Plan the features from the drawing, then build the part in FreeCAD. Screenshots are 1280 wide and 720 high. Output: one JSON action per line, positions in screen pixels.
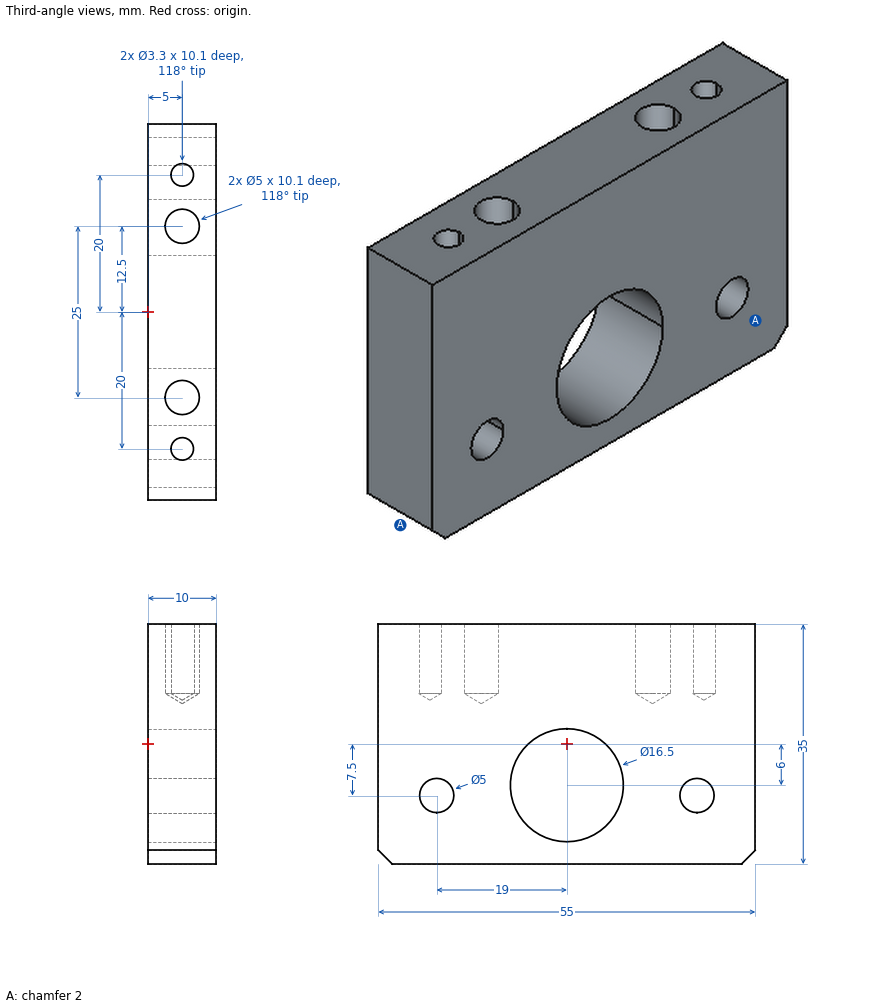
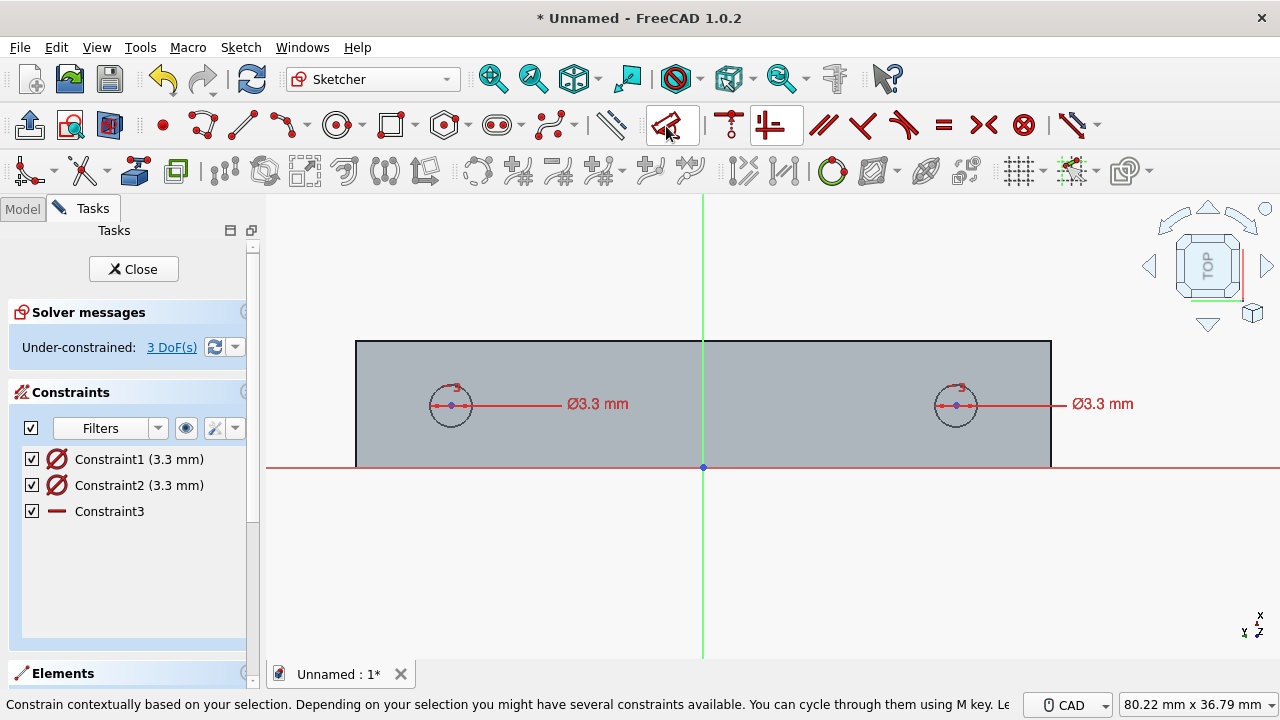
{"action": "left_click", "coordinate": [451, 406]}
{"action": "left_click", "coordinate": [417, 437]}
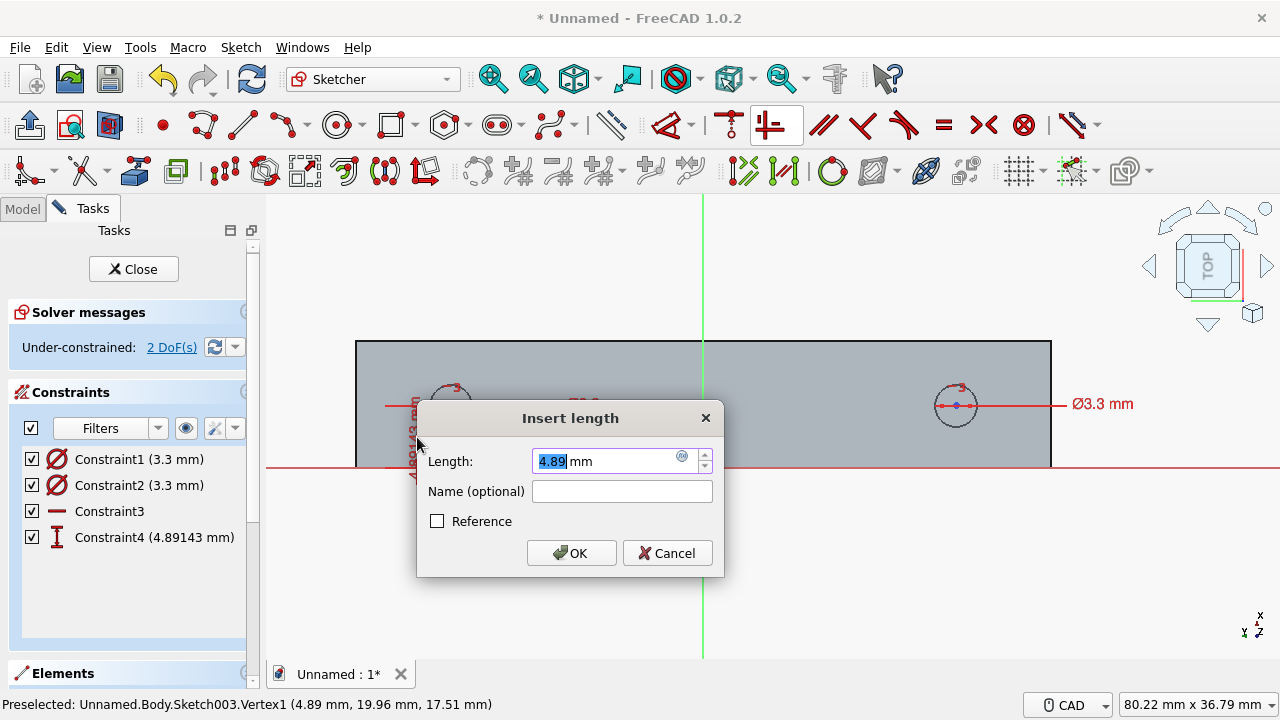
{"action": "type", "text": "5"}
{"action": "key", "text": "Return"}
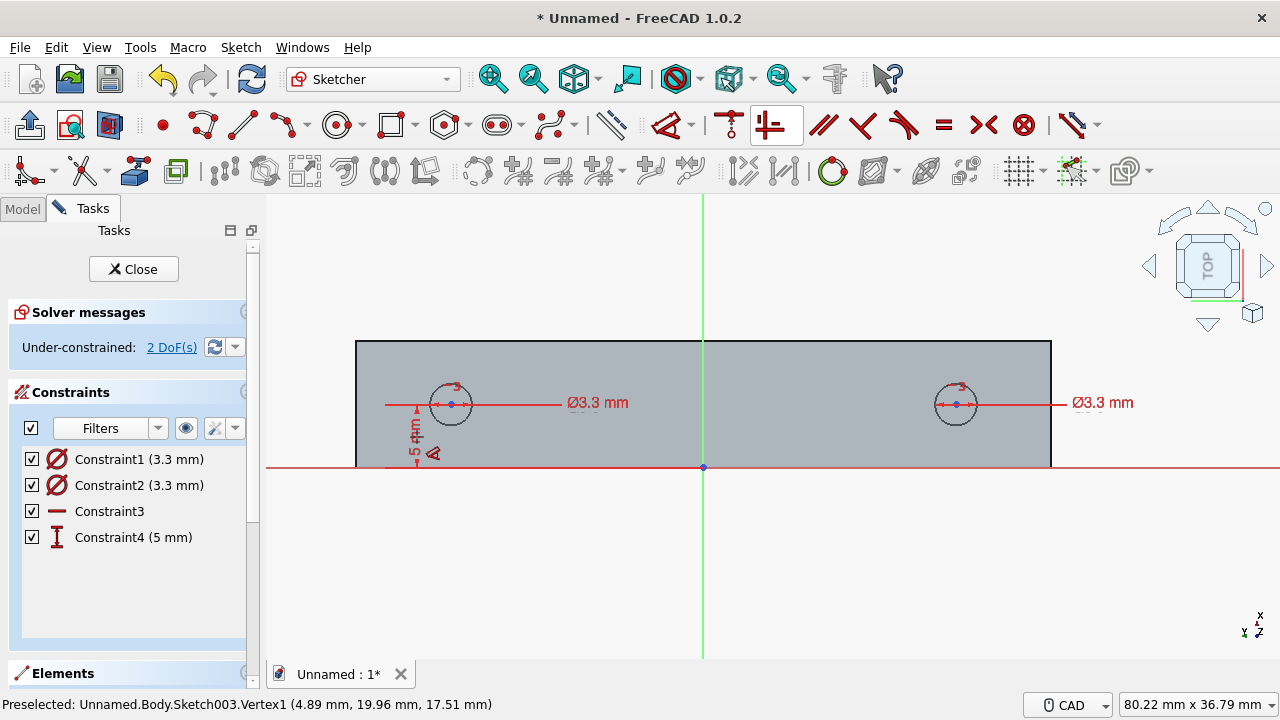
{"action": "left_click", "coordinate": [451, 405]}
{"action": "left_click", "coordinate": [577, 502]}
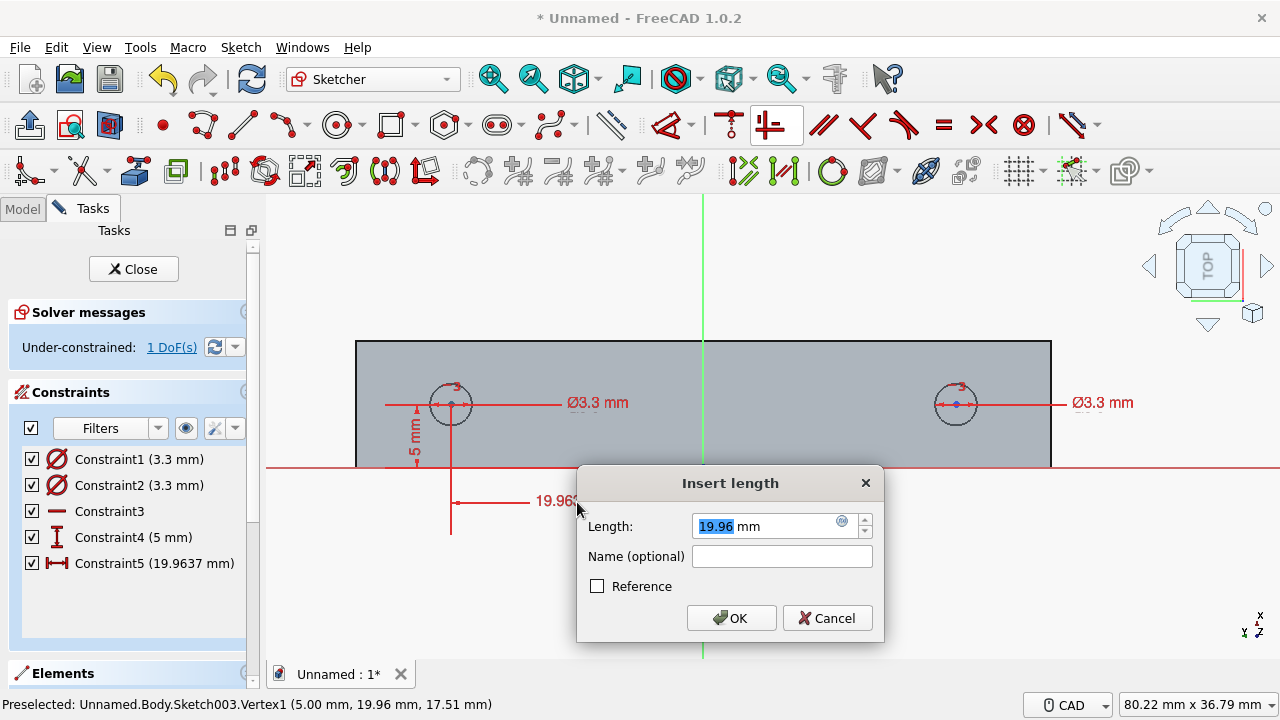
{"action": "type", "text": "20"}
{"action": "key", "text": "Return"}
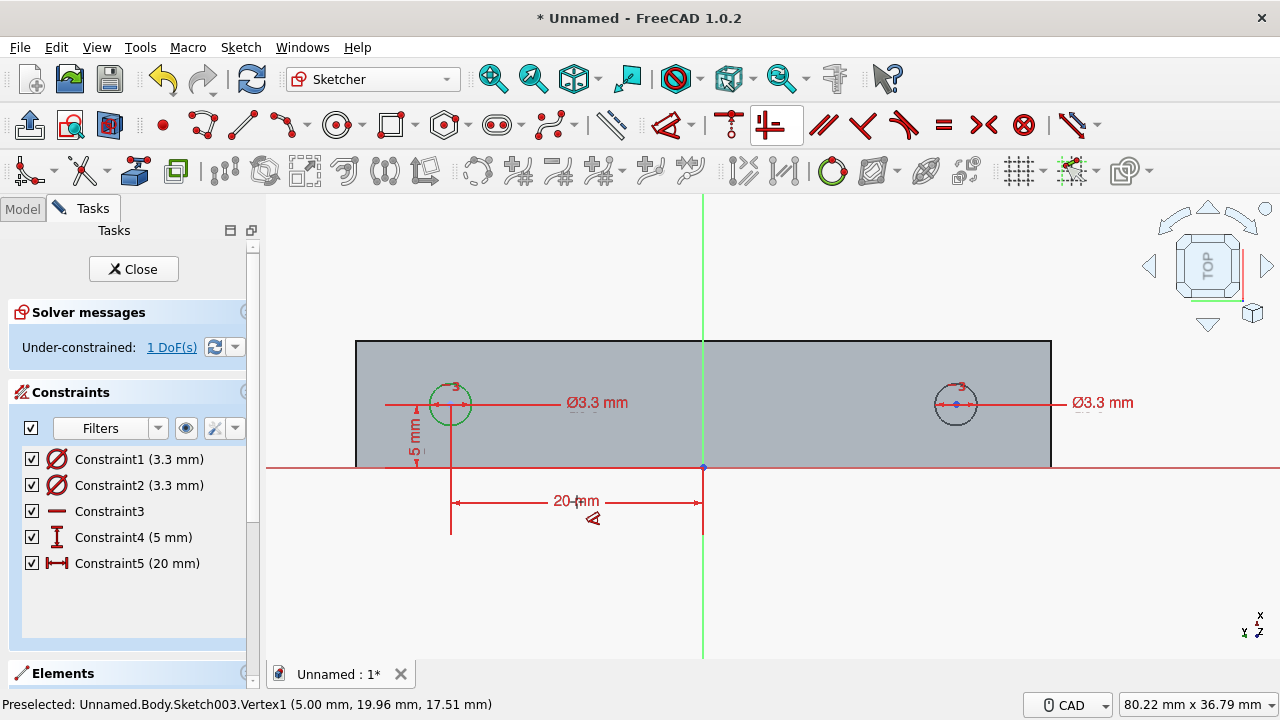
{"action": "left_click", "coordinate": [956, 405]}
{"action": "left_click", "coordinate": [830, 502]}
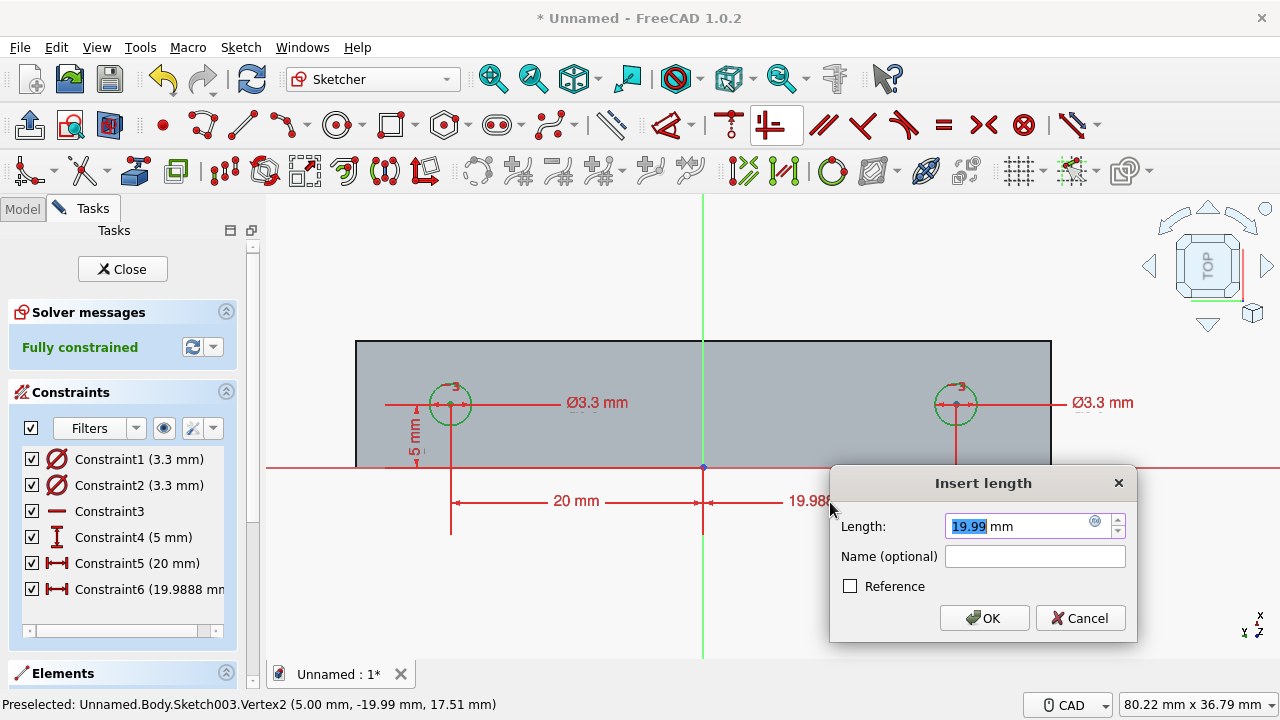
{"action": "type", "text": "20"}
{"action": "key", "text": "Return"}
{"action": "key", "text": "Escape"}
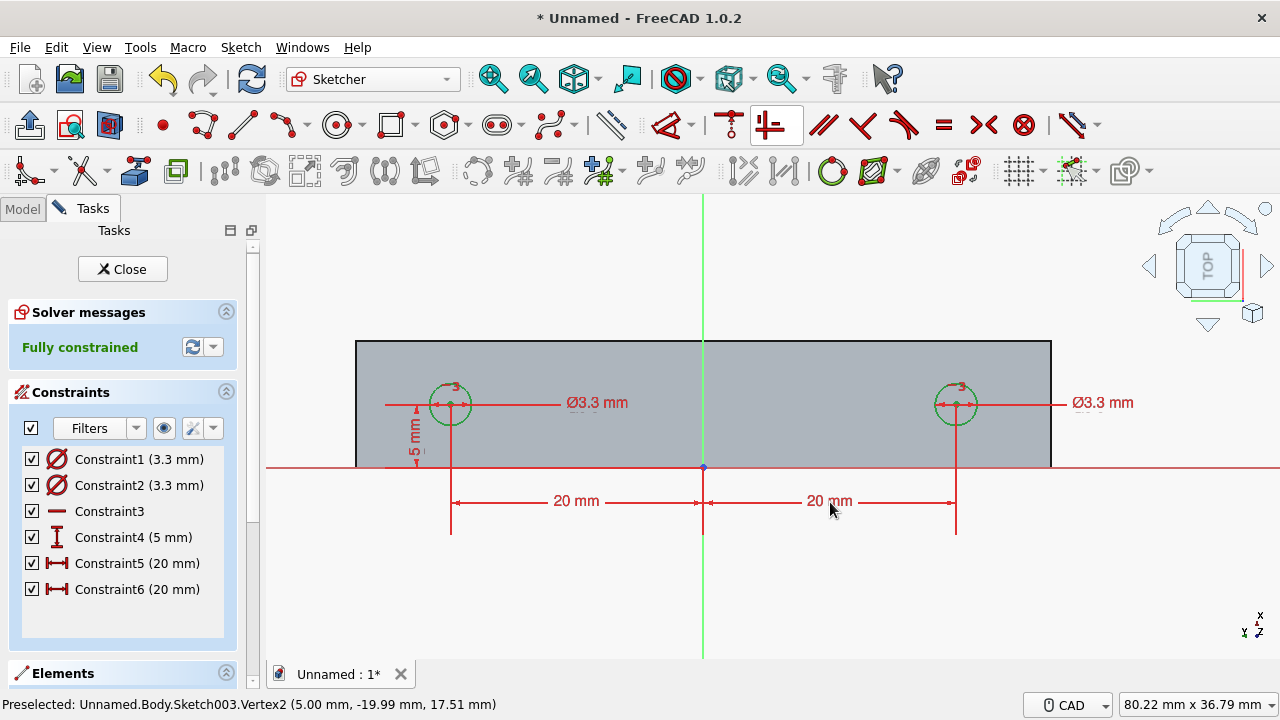
{"action": "left_click", "coordinate": [123, 269]}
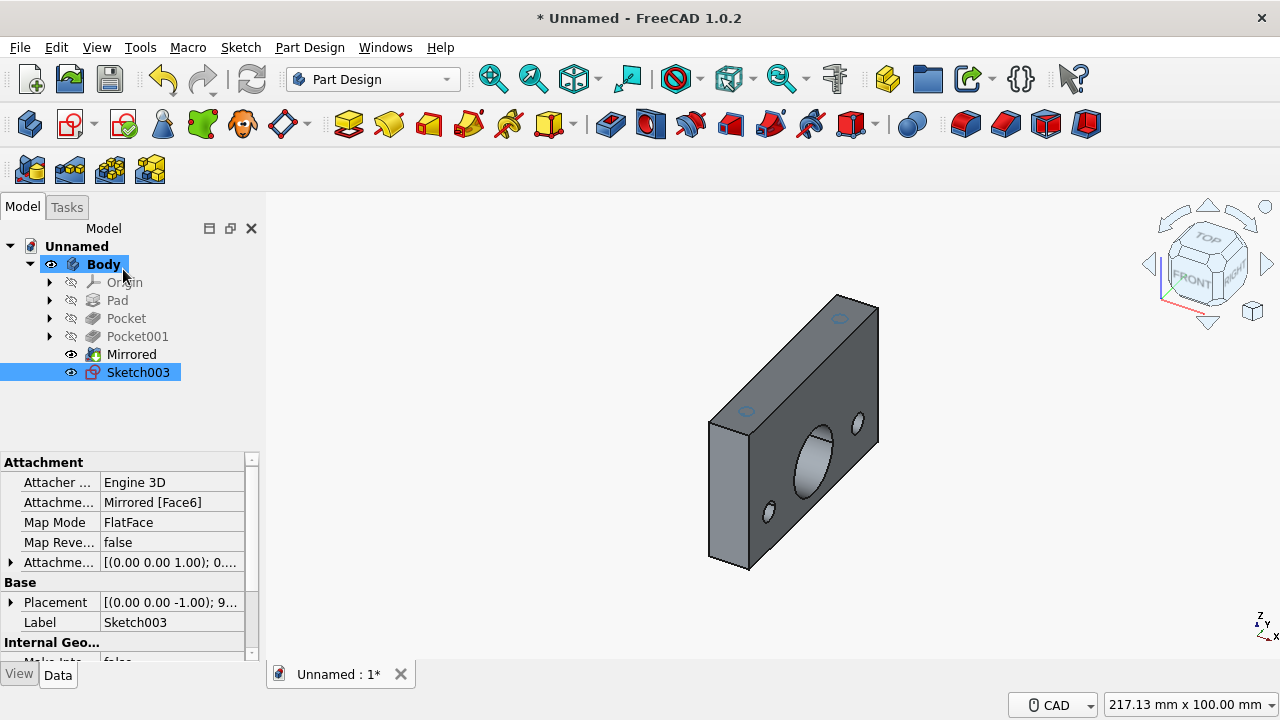
{"action": "left_click", "coordinate": [652, 124]}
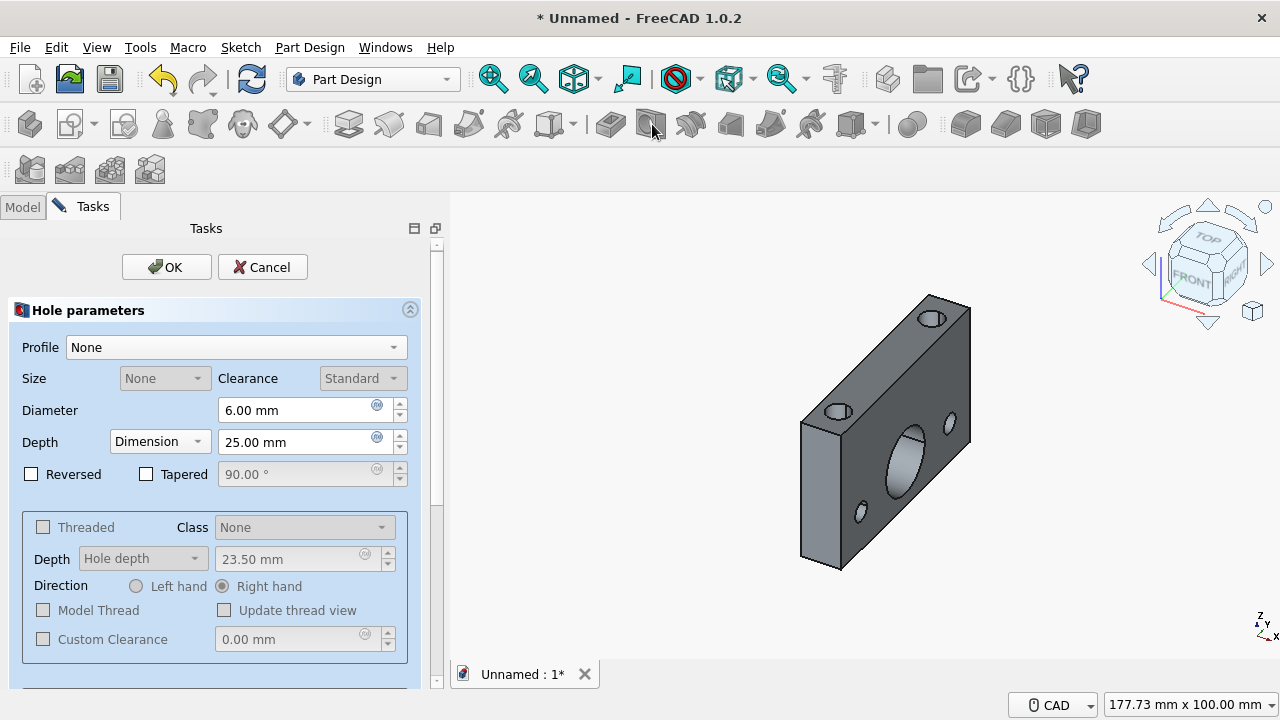
{"action": "triple_click", "coordinate": [305, 410]}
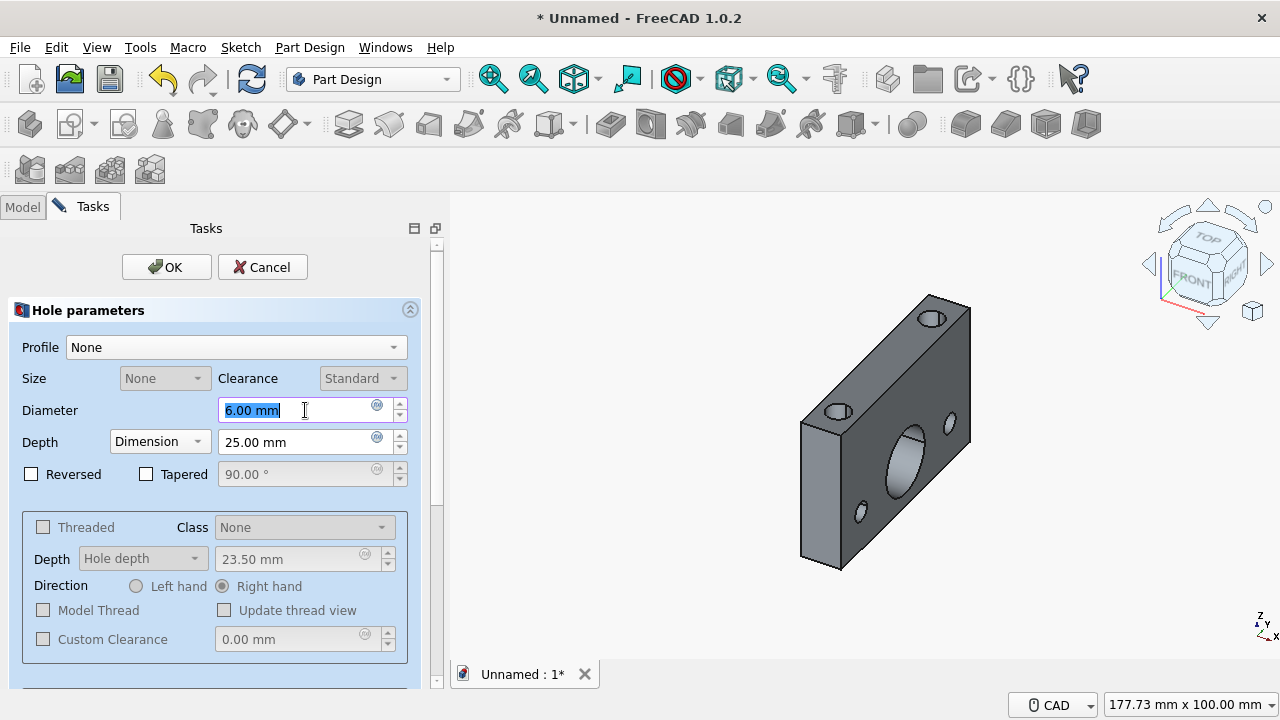
{"action": "type", "text": "3.3"}
{"action": "key", "text": "Tab"}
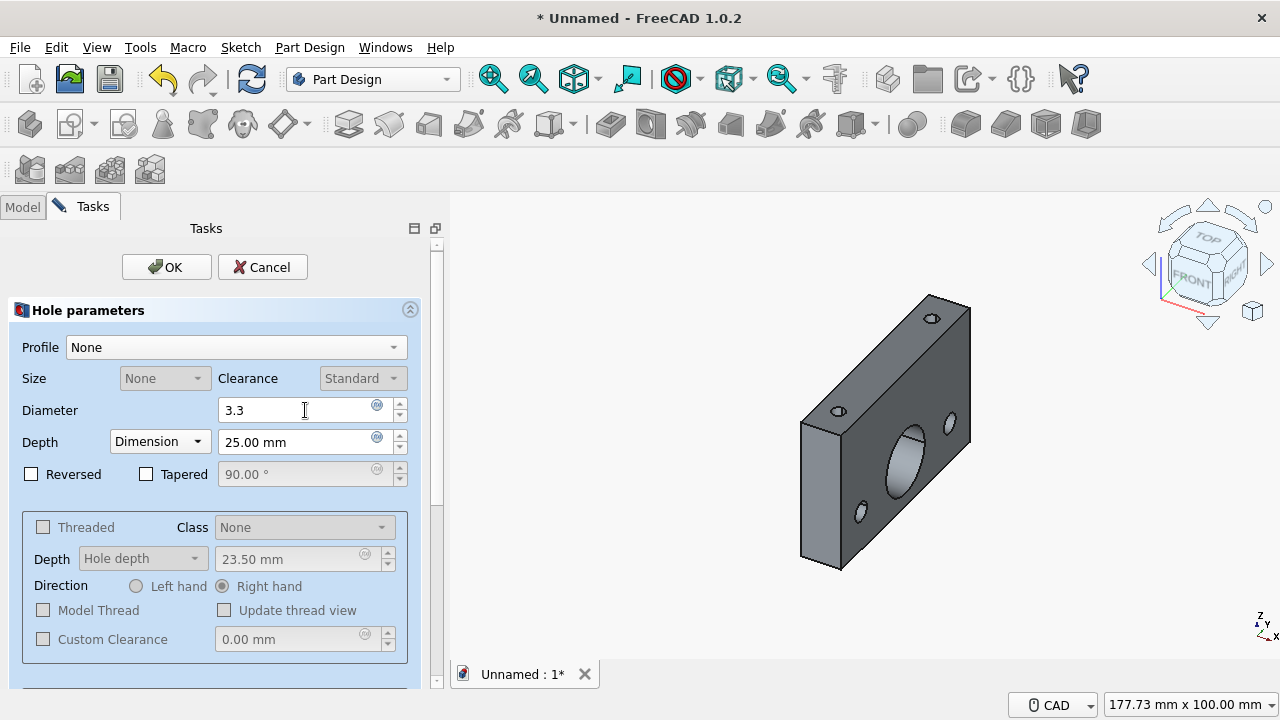
{"action": "triple_click", "coordinate": [305, 442]}